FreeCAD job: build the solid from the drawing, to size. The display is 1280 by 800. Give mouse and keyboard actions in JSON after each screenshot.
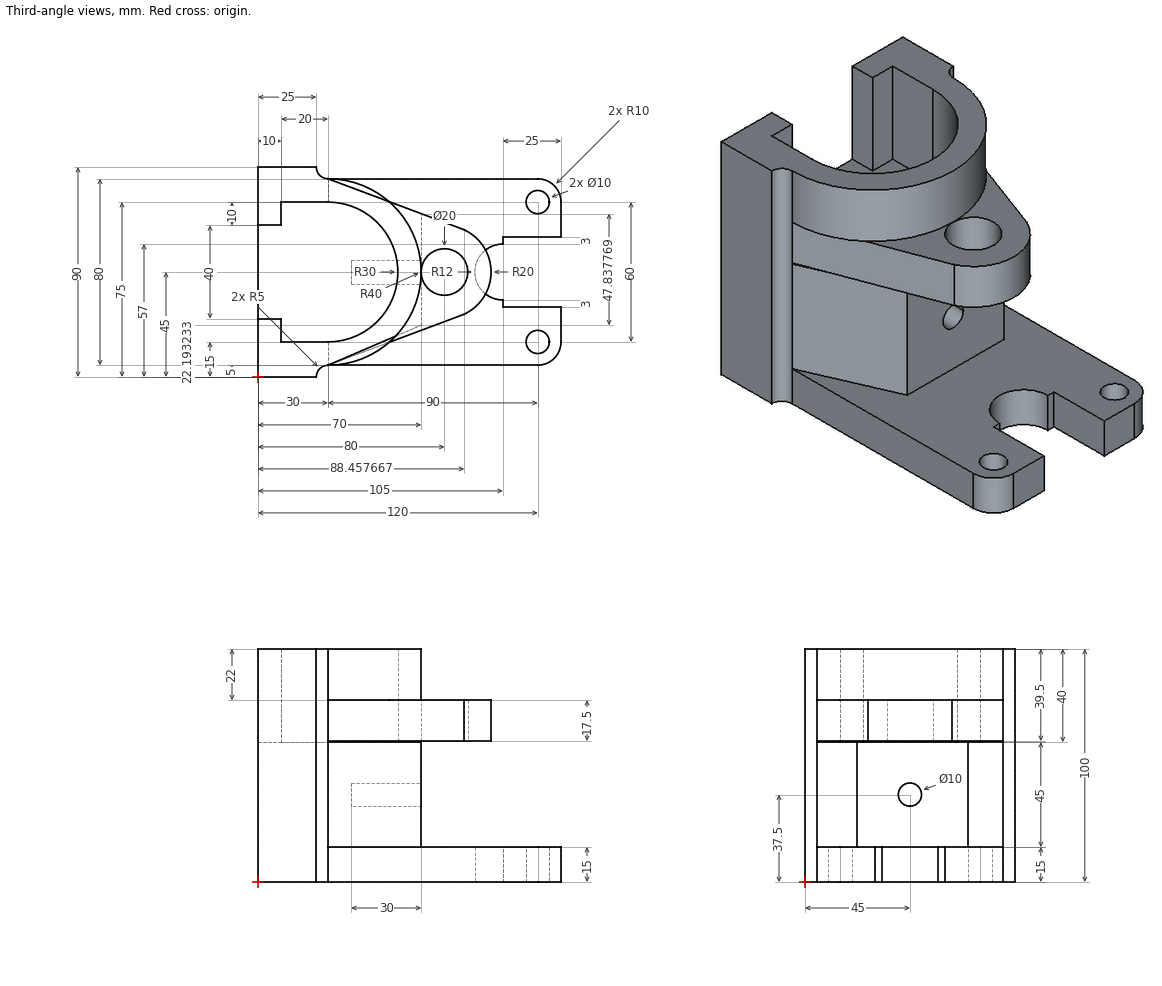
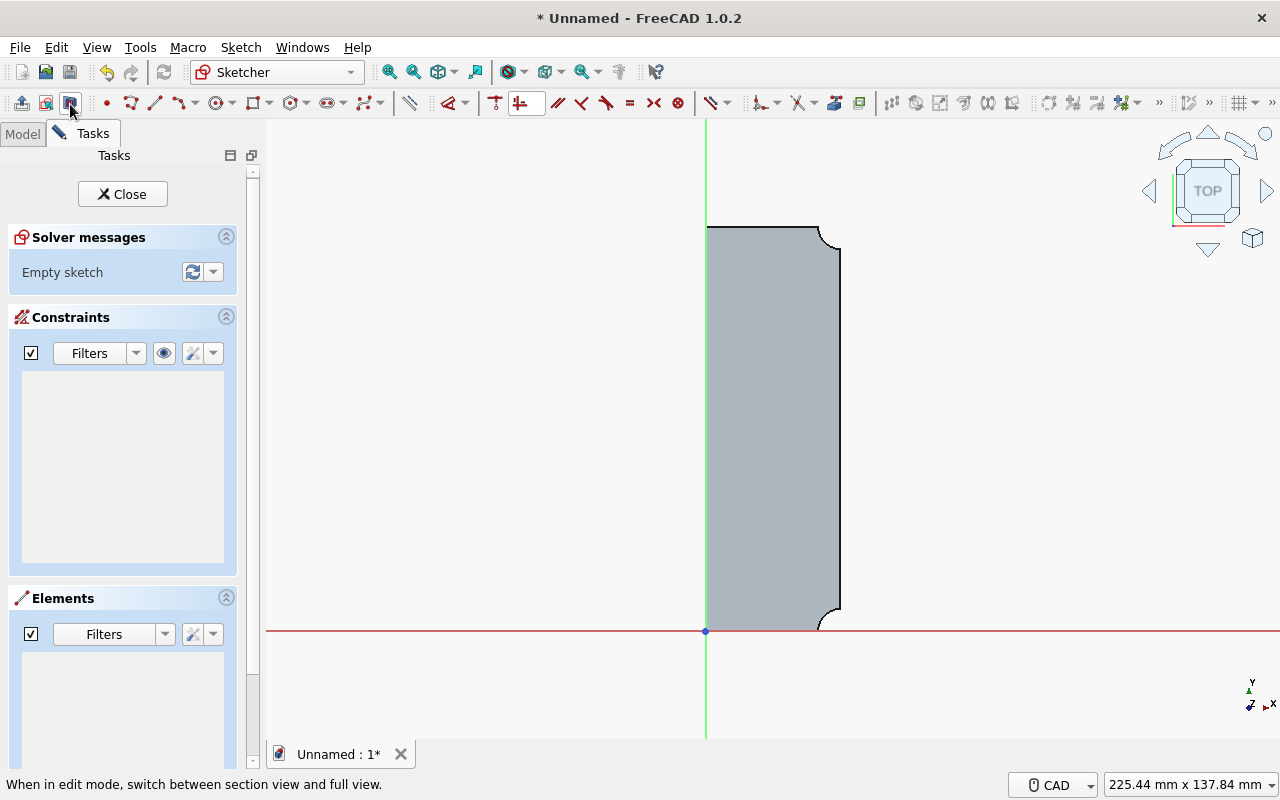
{"action": "scroll", "coordinate": [294, 406], "scroll_direction": "down", "scroll_amount": 2}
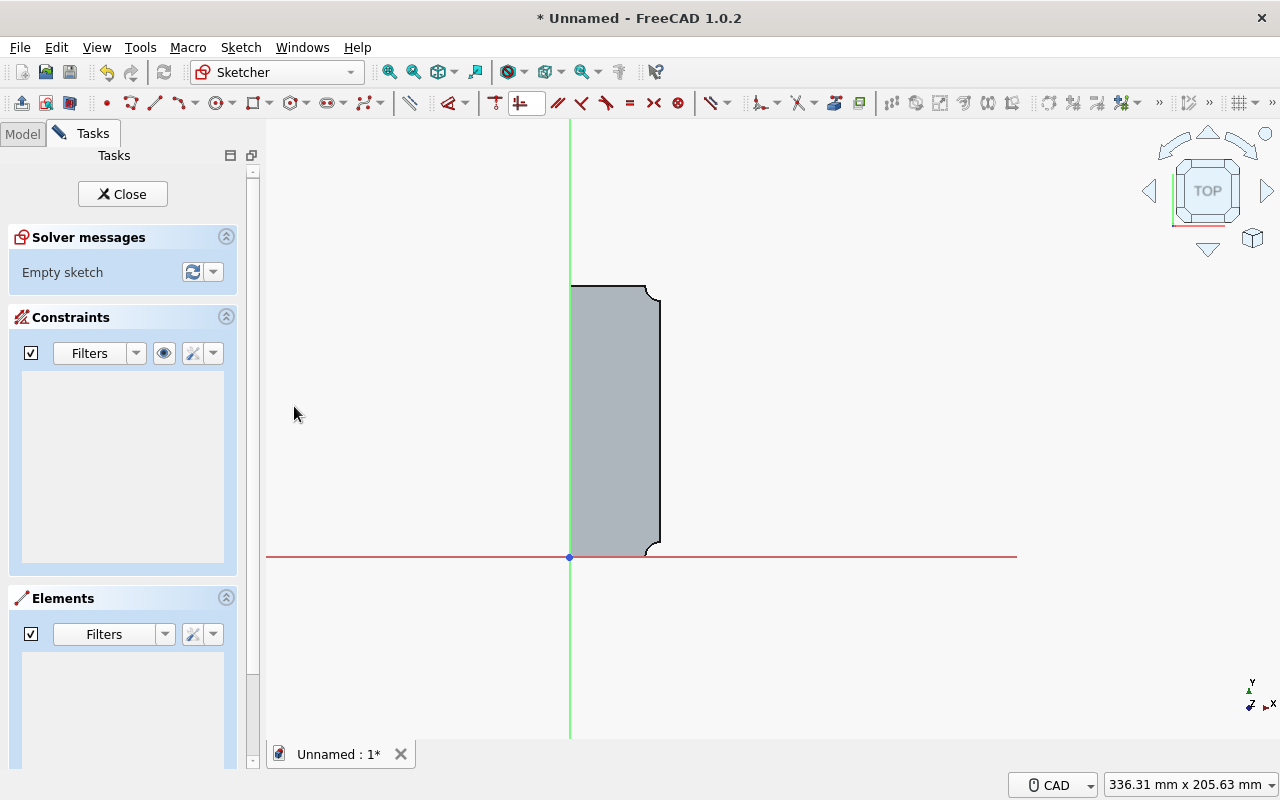
{"action": "scroll", "coordinate": [891, 429], "scroll_direction": "up", "scroll_amount": 2}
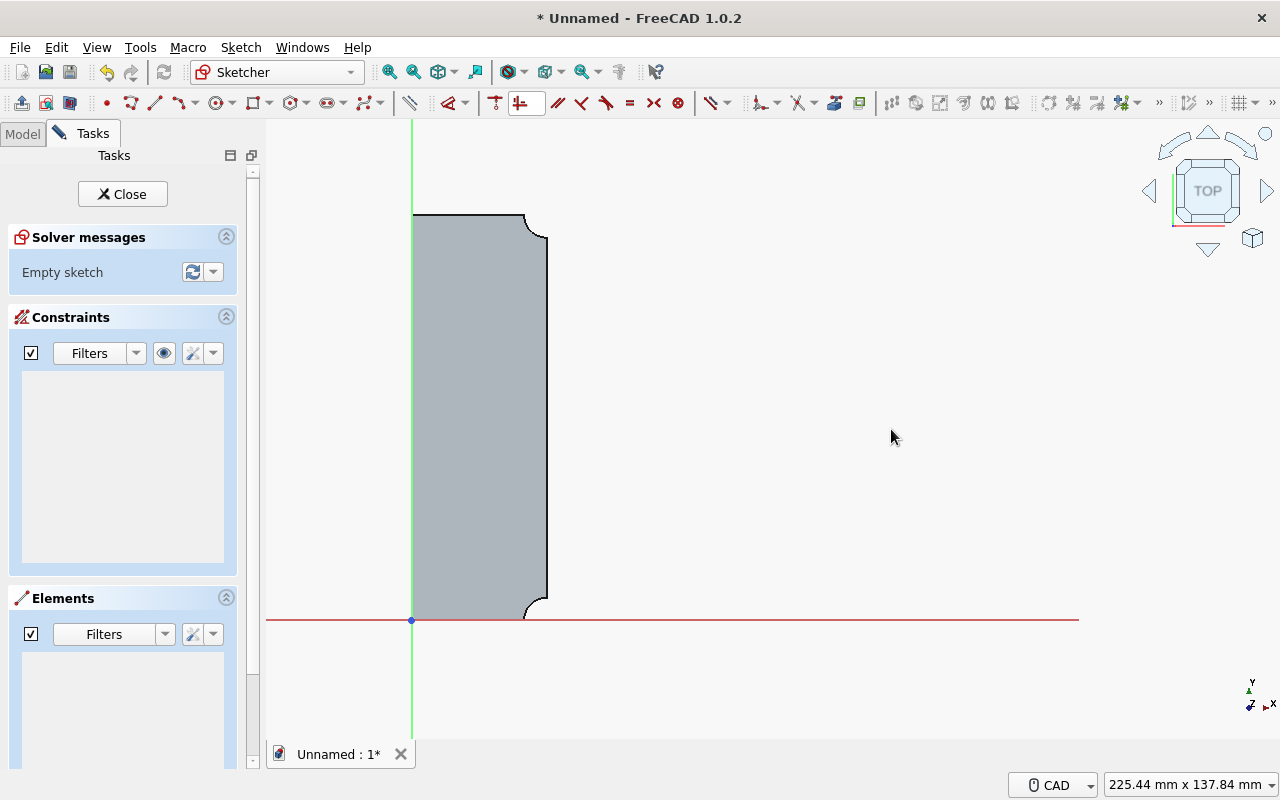
{"action": "left_click", "coordinate": [156, 104]}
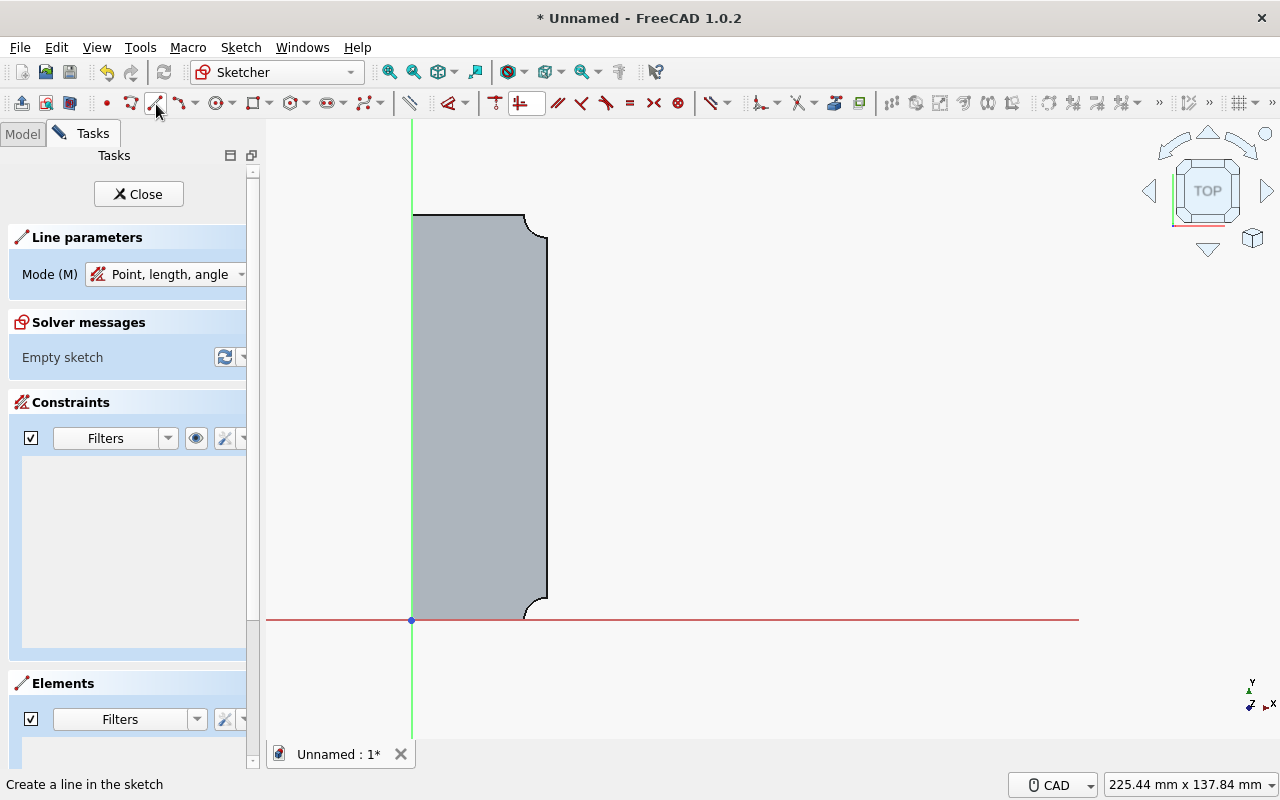
{"action": "left_click", "coordinate": [996, 283]}
{"action": "left_click", "coordinate": [996, 553]}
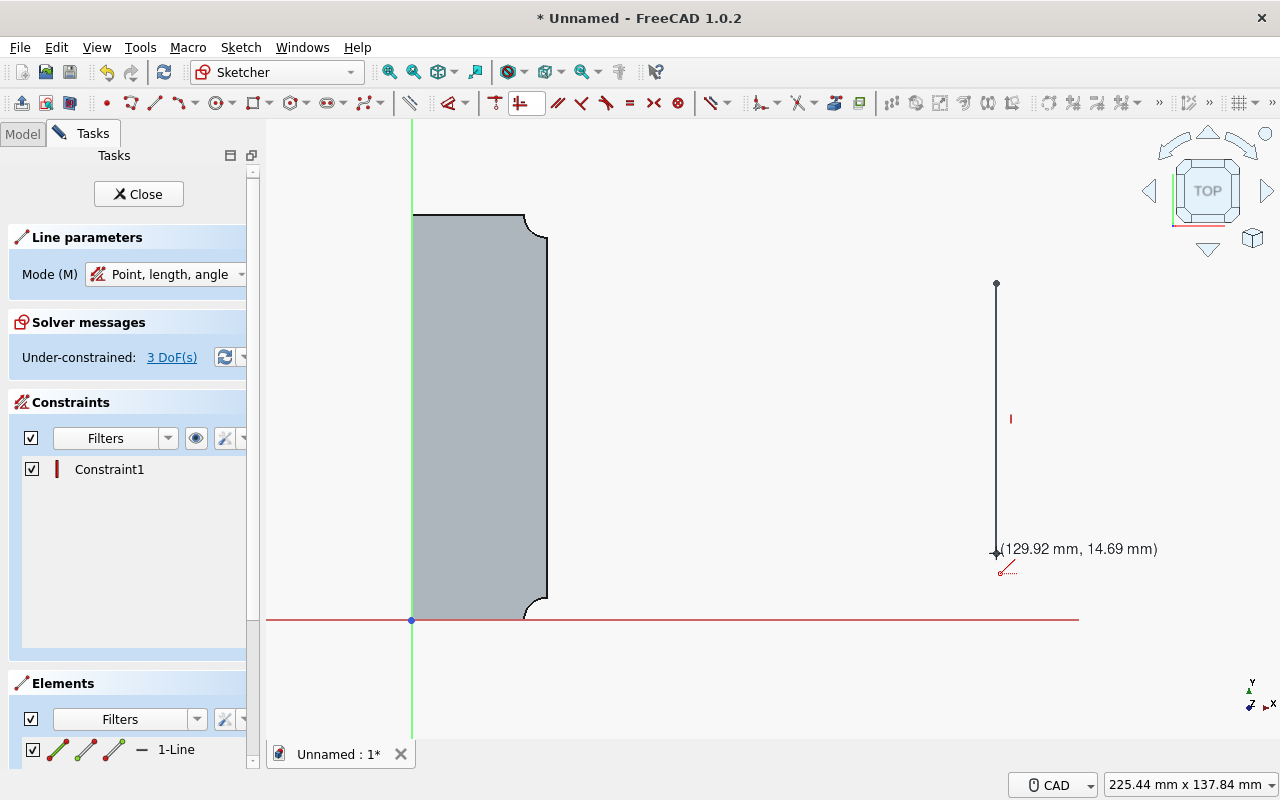
{"action": "left_click", "coordinate": [132, 104]}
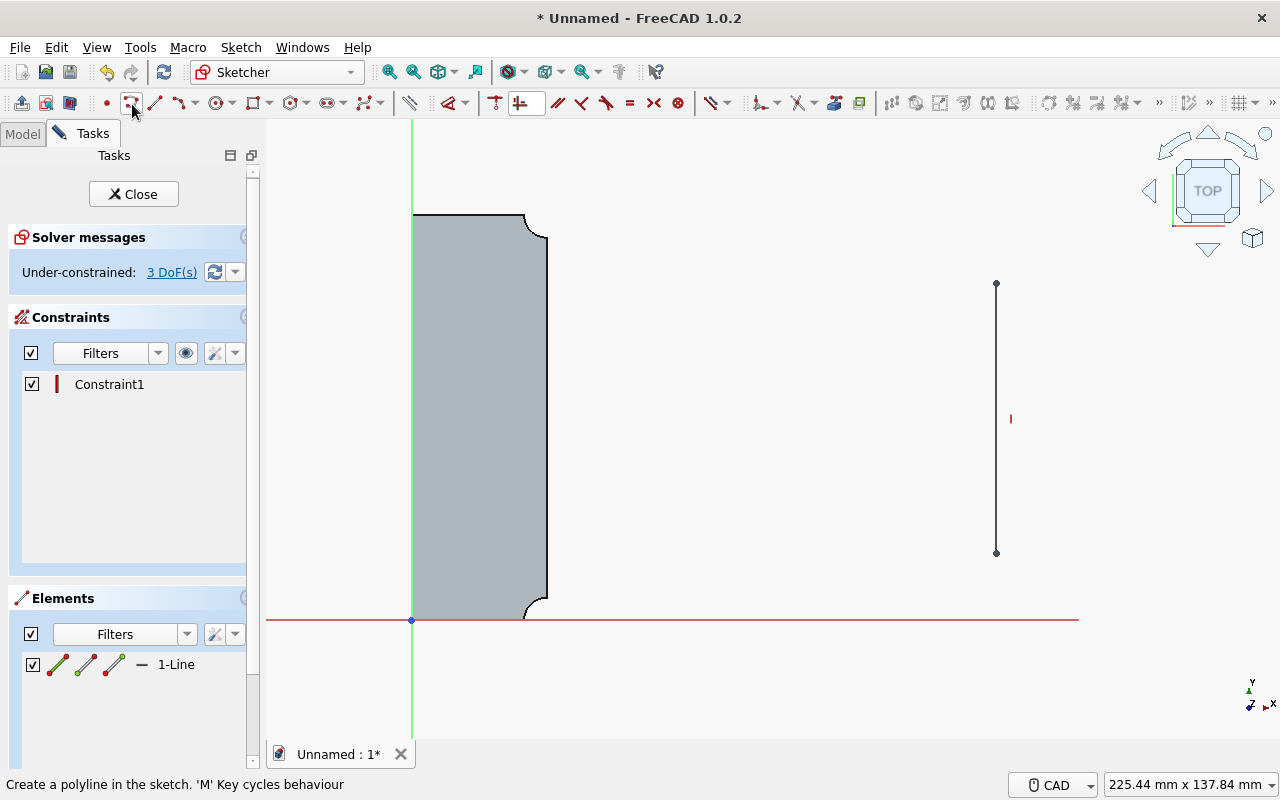
{"action": "left_click", "coordinate": [951, 598]}
{"action": "left_click", "coordinate": [547, 598]}
{"action": "left_click", "coordinate": [547, 238]}
{"action": "left_click", "coordinate": [951, 238]}
{"action": "right_click", "coordinate": [951, 238]}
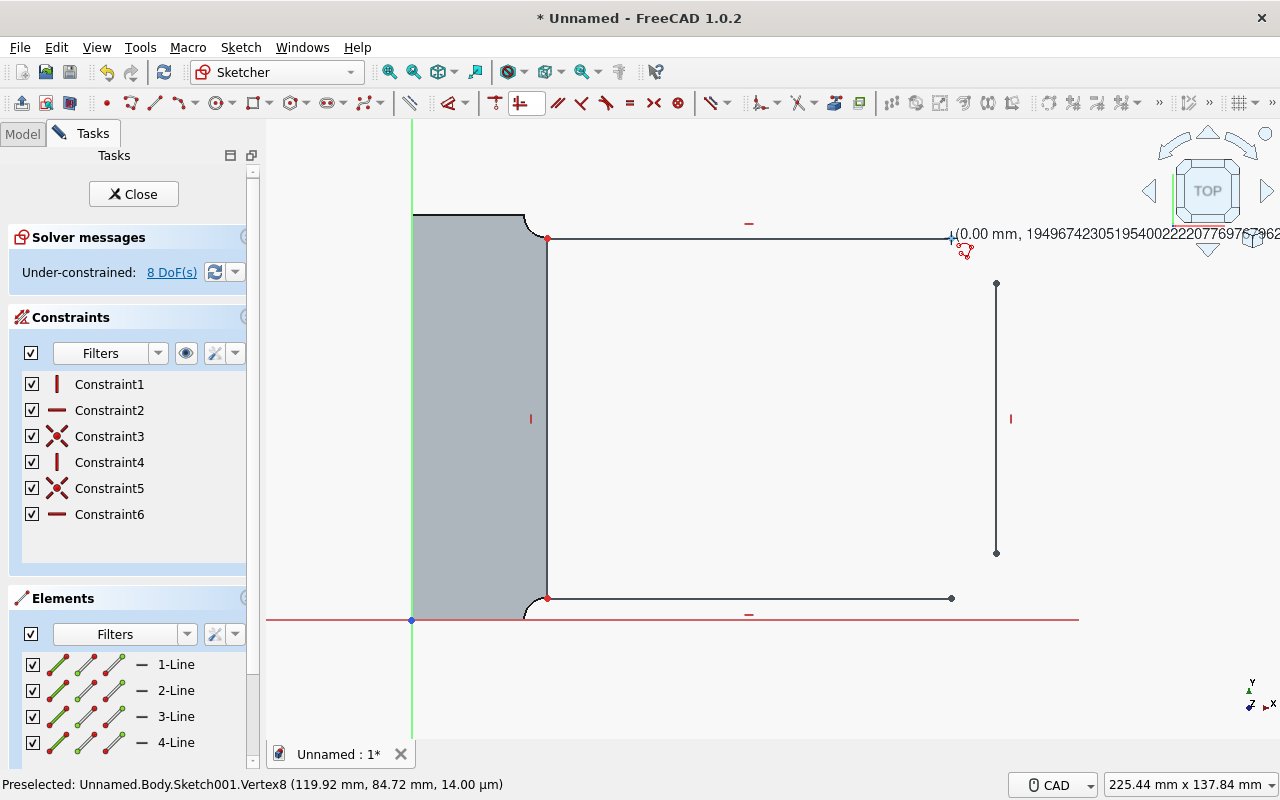
{"action": "key", "text": "g 3 a"}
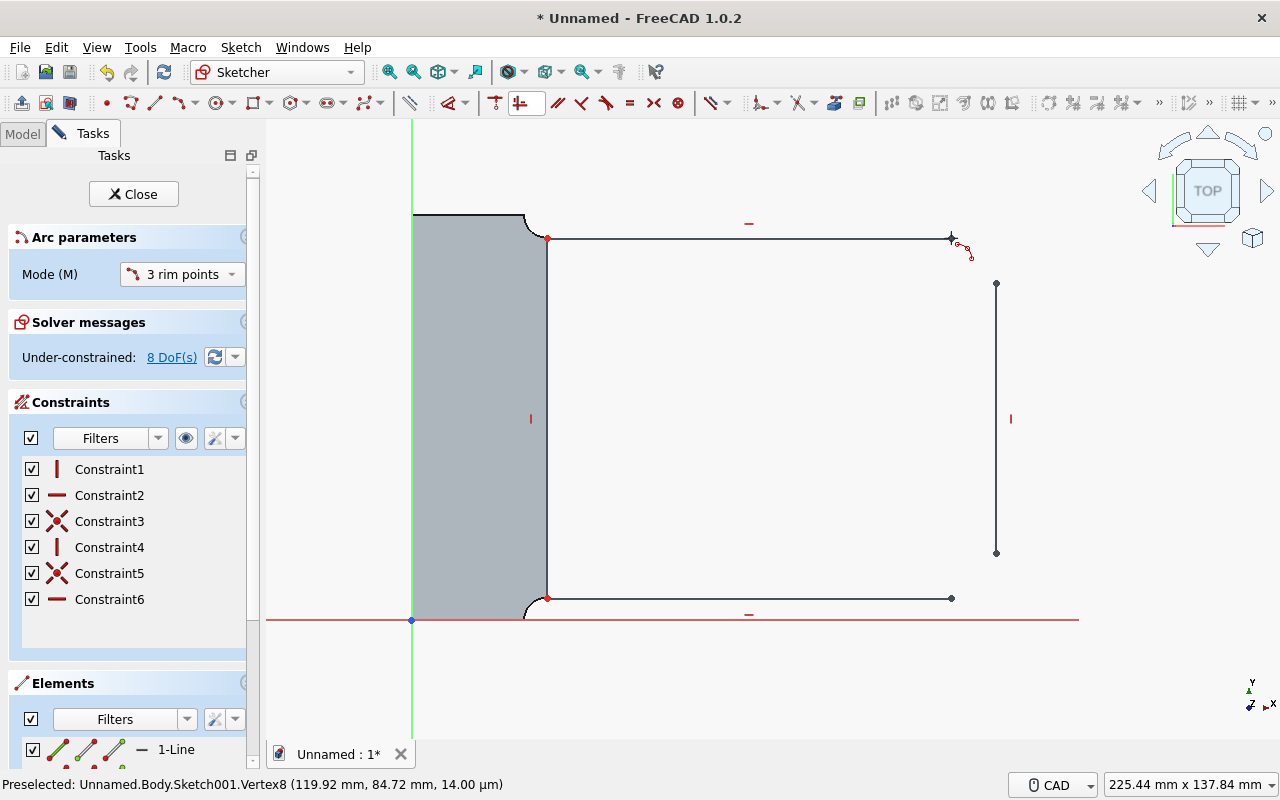
{"action": "left_click", "coordinate": [996, 554]}
{"action": "left_click", "coordinate": [951, 599]}
{"action": "left_click", "coordinate": [983, 584]}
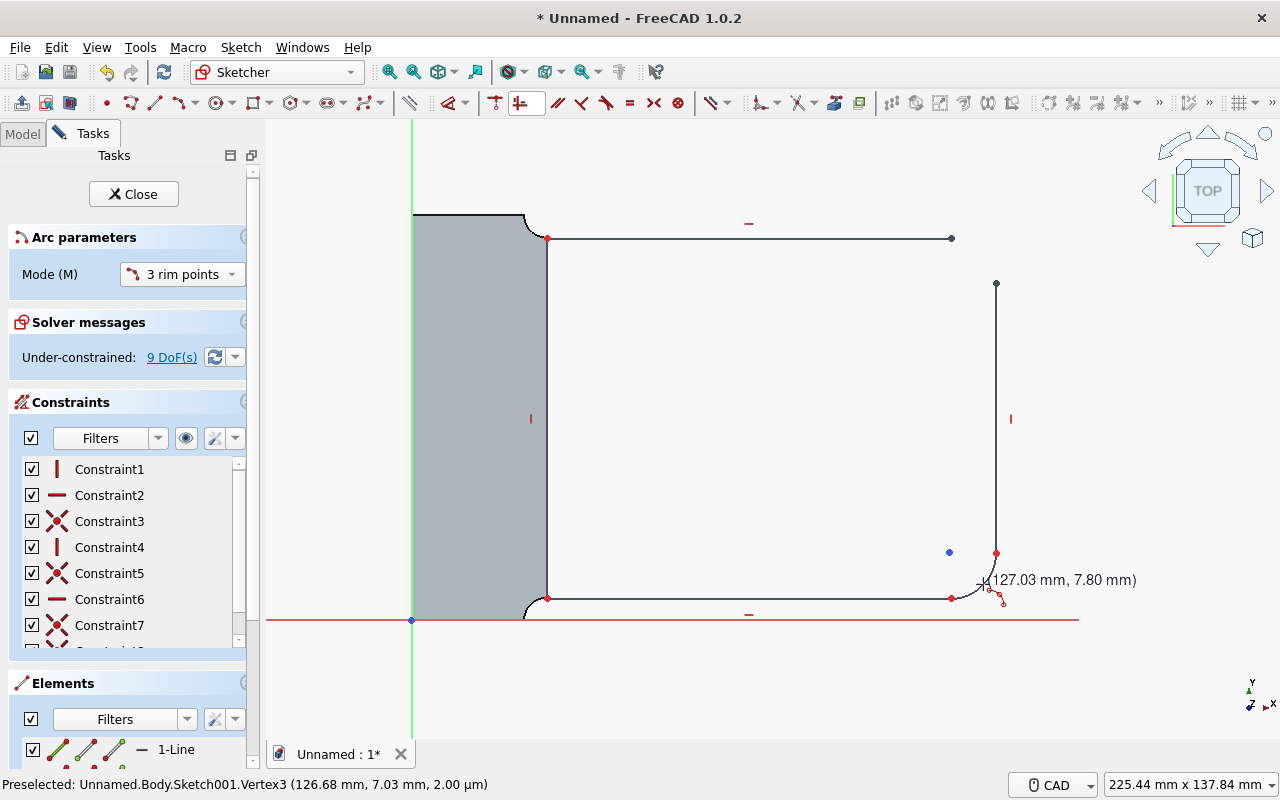
{"action": "left_click", "coordinate": [951, 239]}
{"action": "left_click", "coordinate": [996, 284]}
{"action": "left_click", "coordinate": [983, 251]}
{"action": "key", "text": "Escape"}